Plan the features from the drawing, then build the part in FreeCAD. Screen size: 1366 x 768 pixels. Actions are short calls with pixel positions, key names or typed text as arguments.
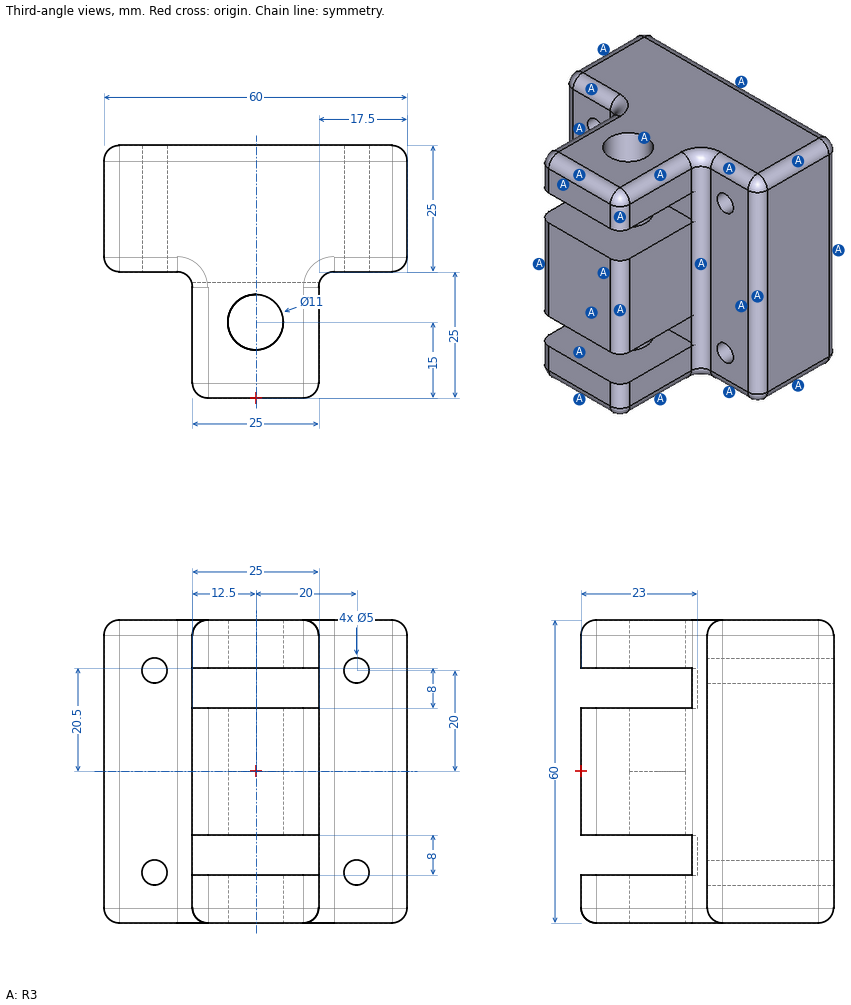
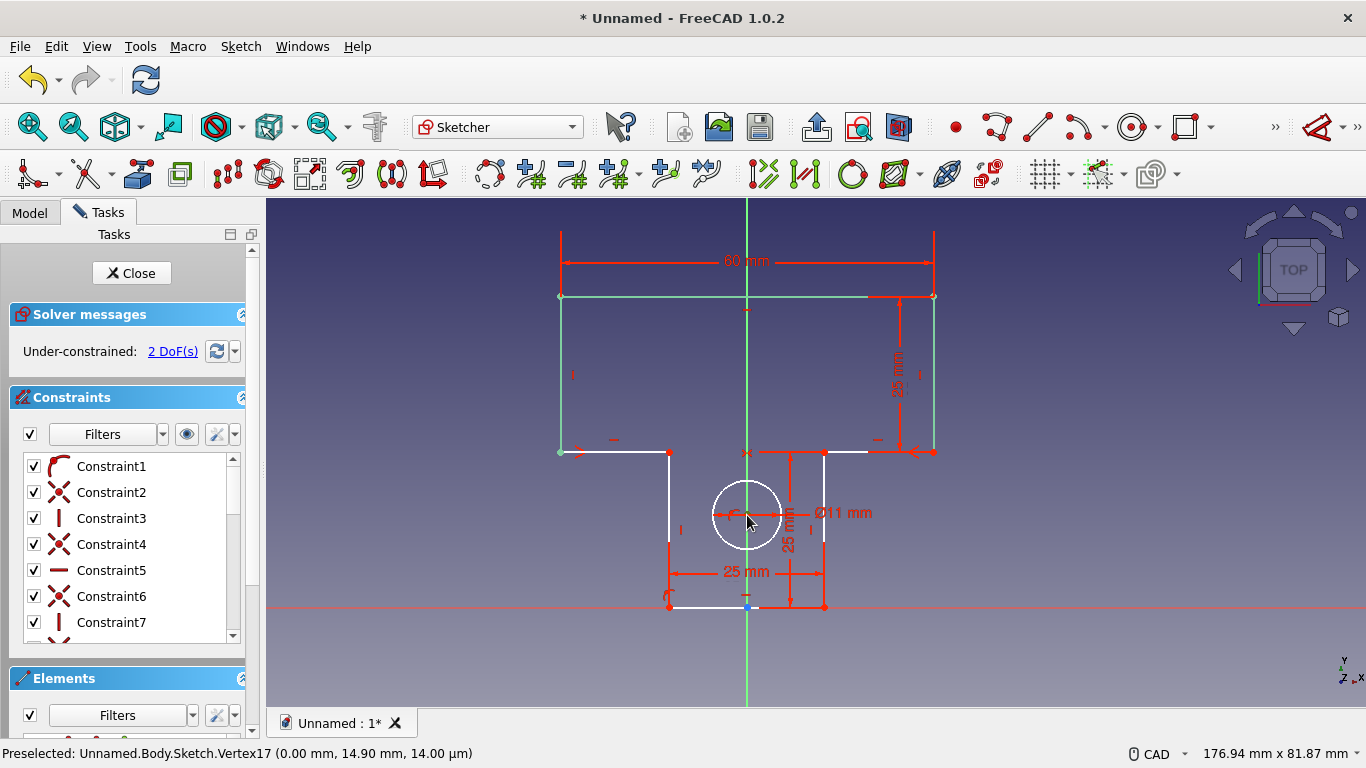
click(1342, 128)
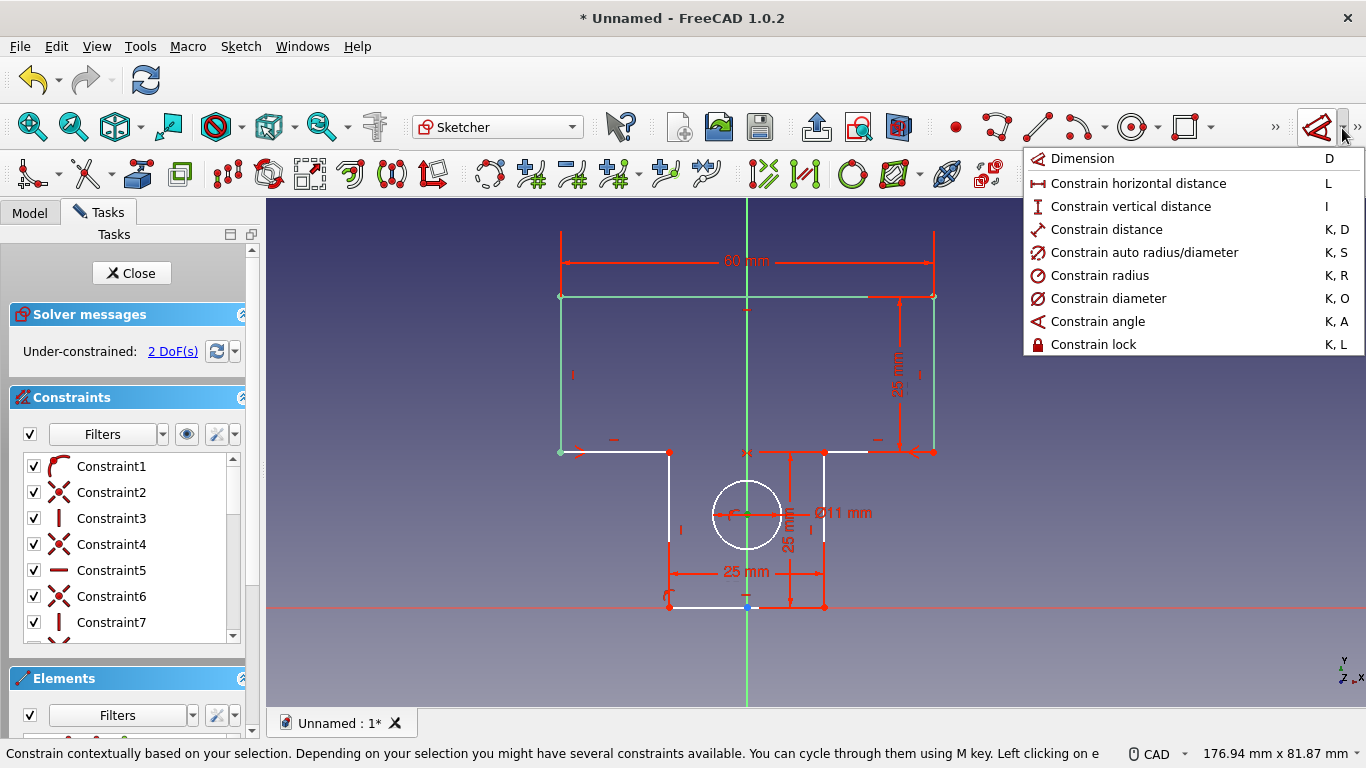
click(1194, 206)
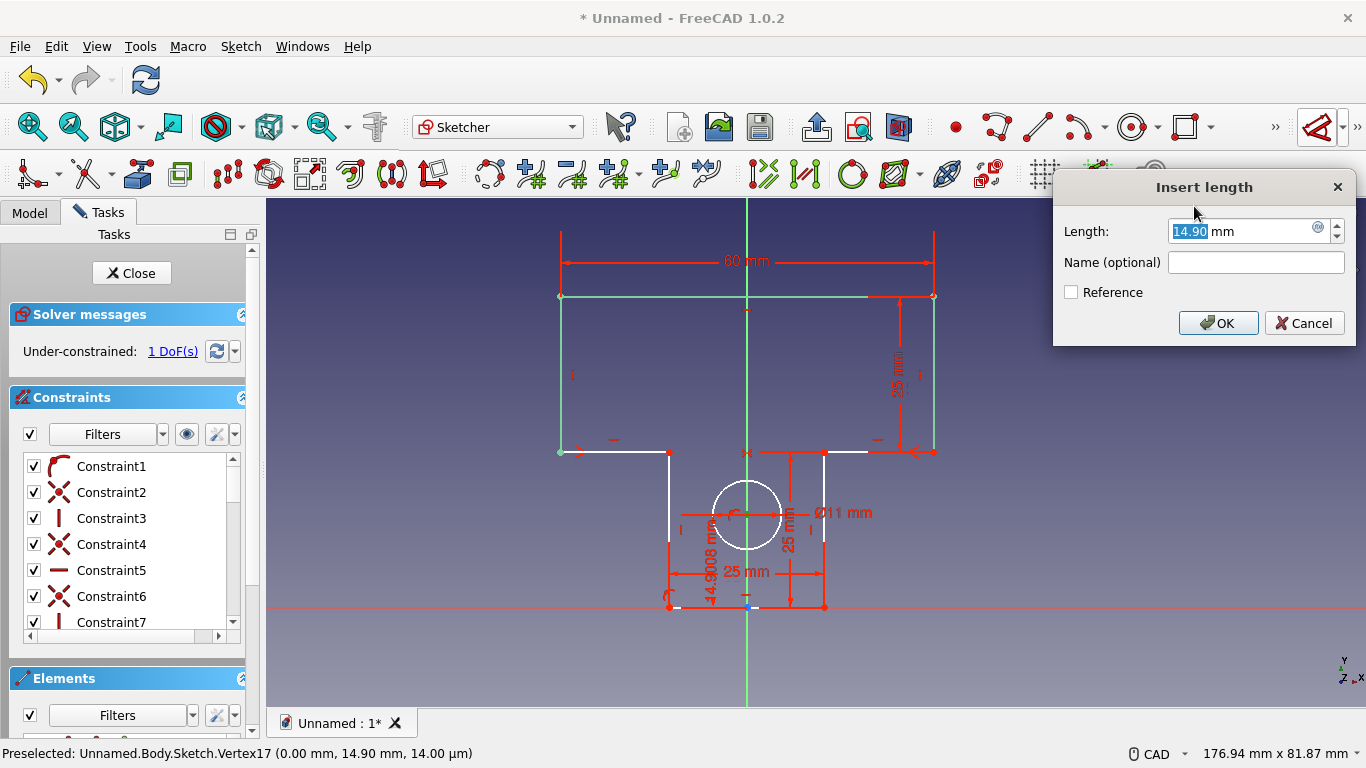
text(15)
key(Return)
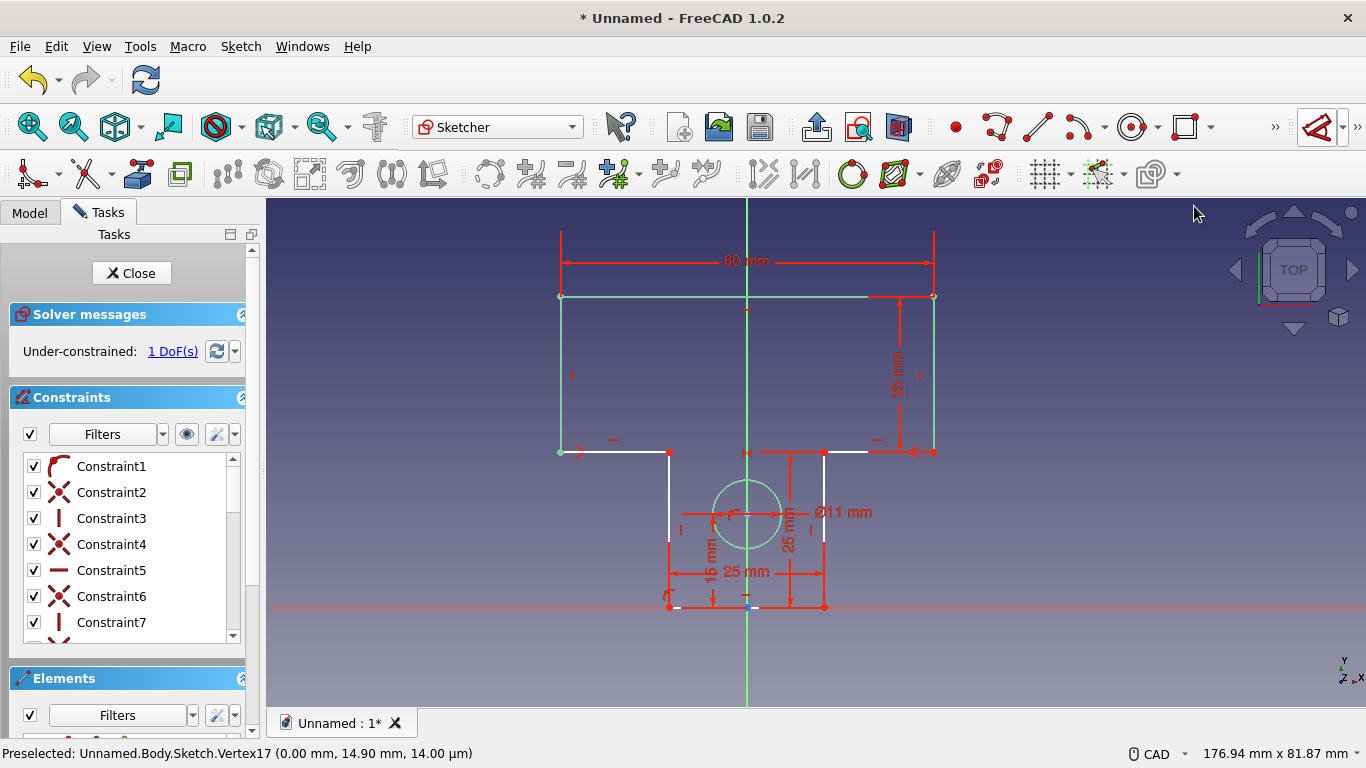
click(857, 452)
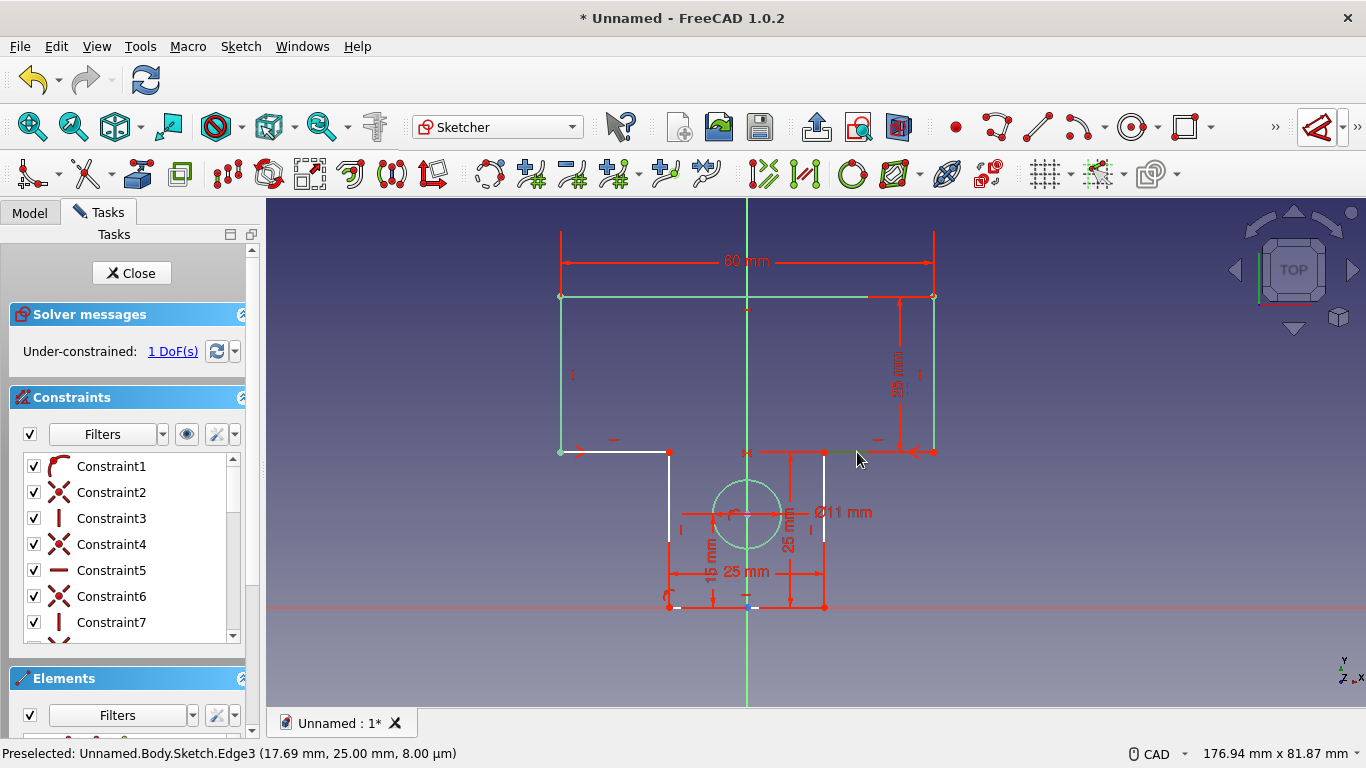
click(1342, 128)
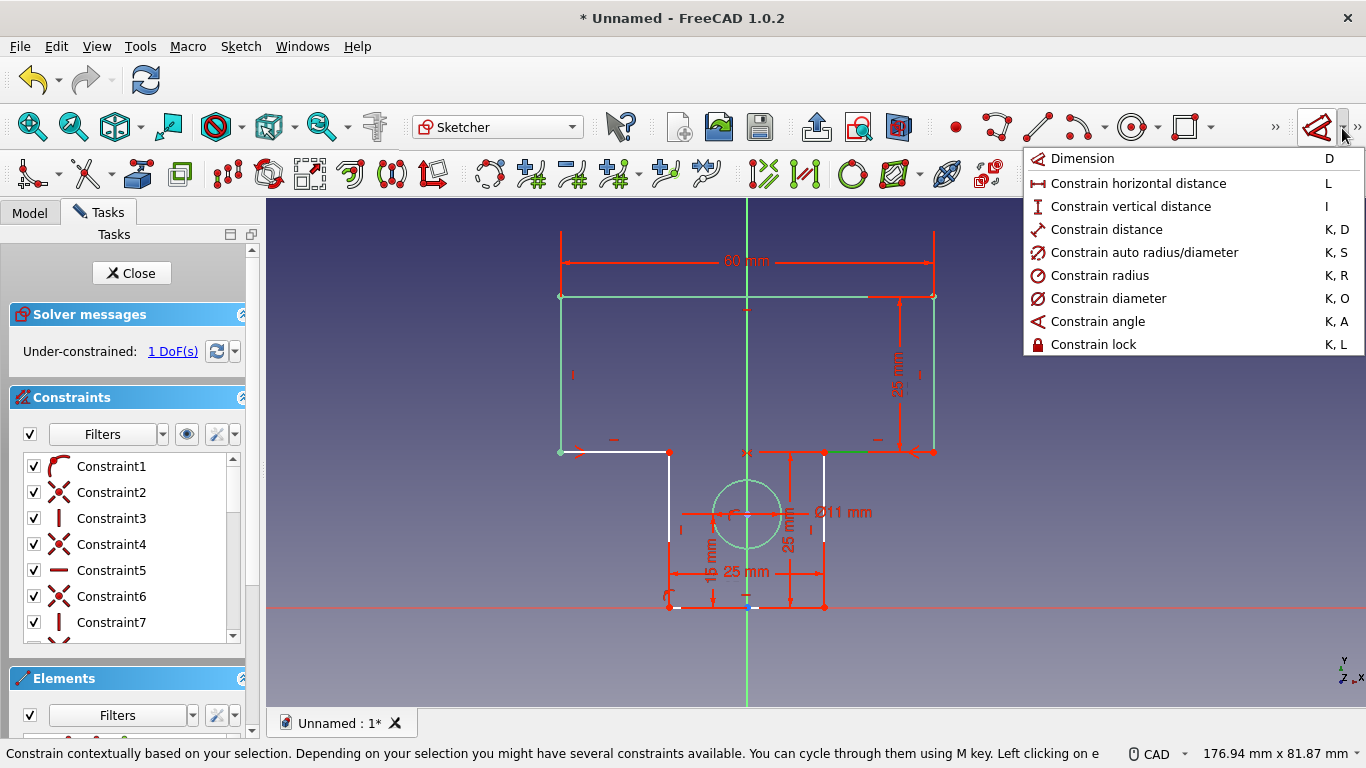
click(1194, 184)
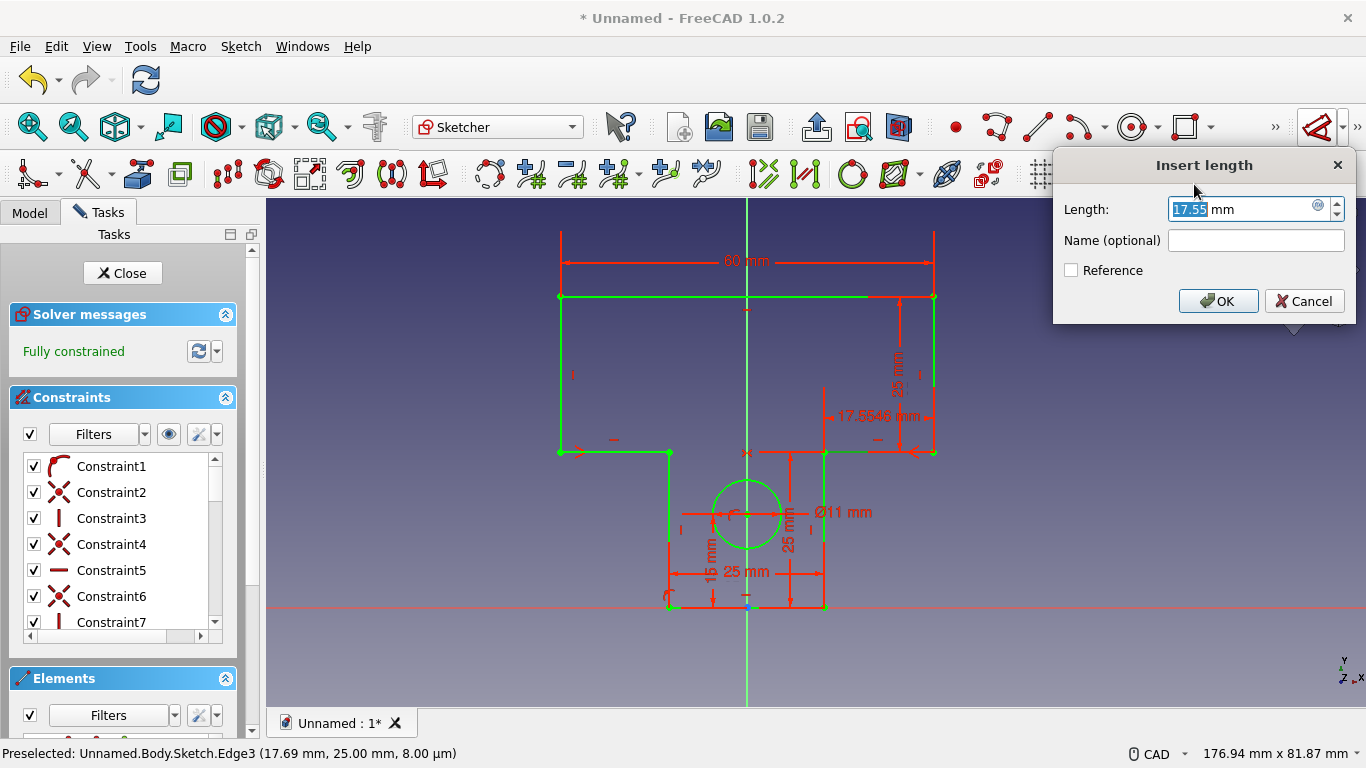
text(17.5)
key(Return)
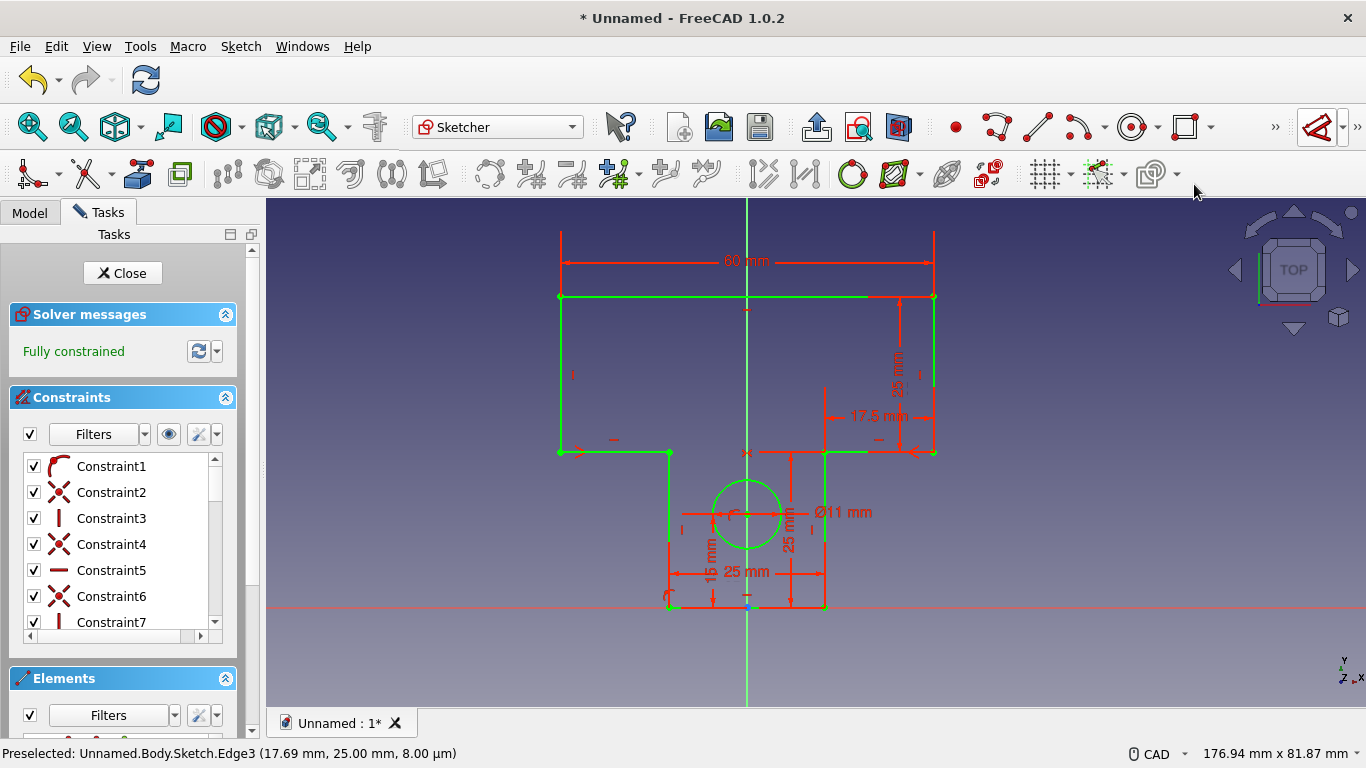
click(123, 273)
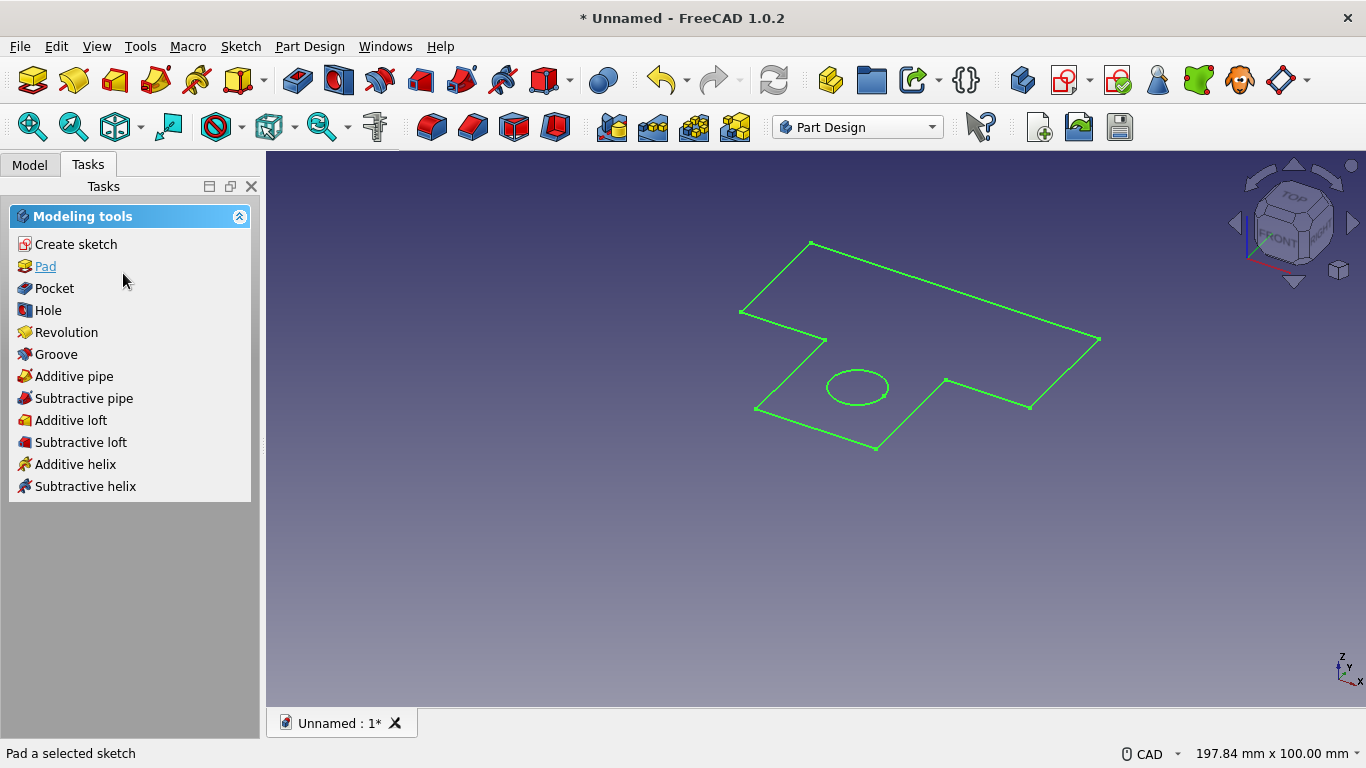
click(33, 80)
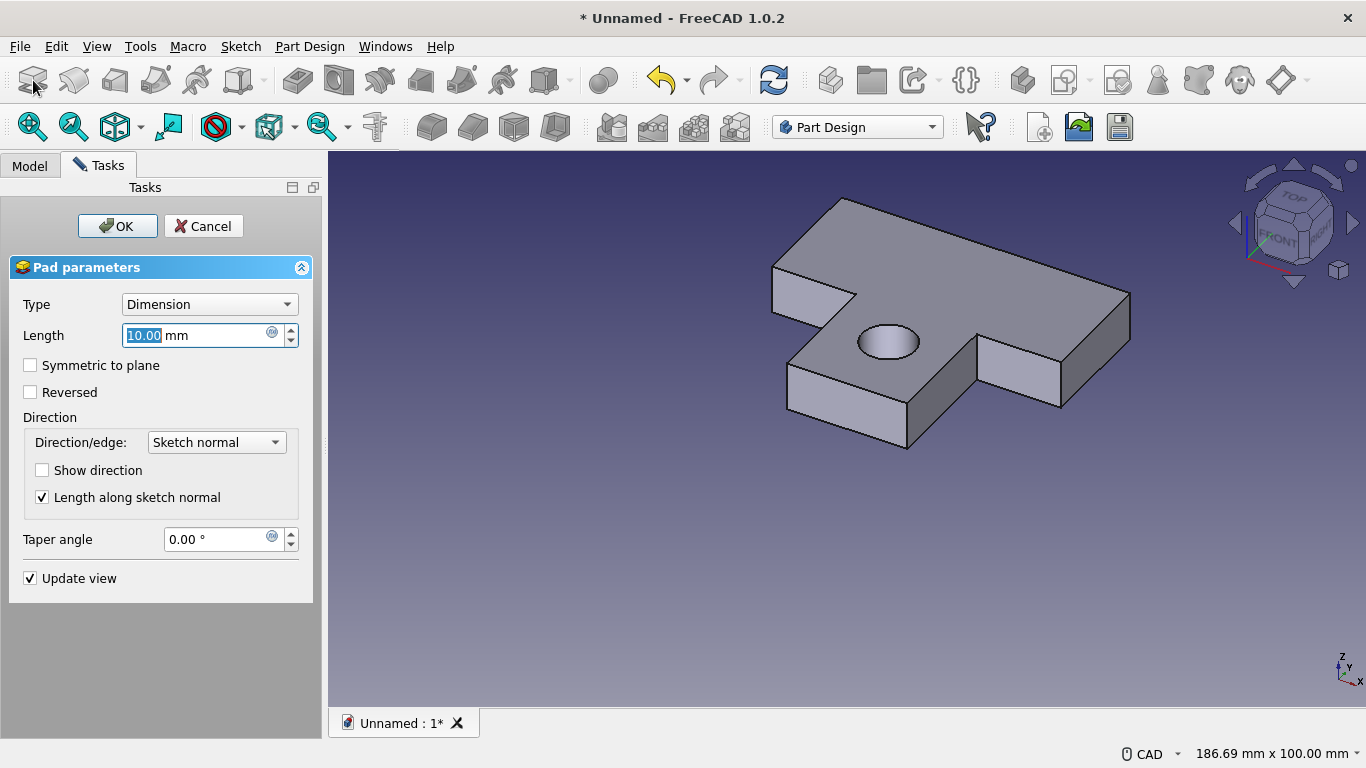
text(60)
key(Tab)